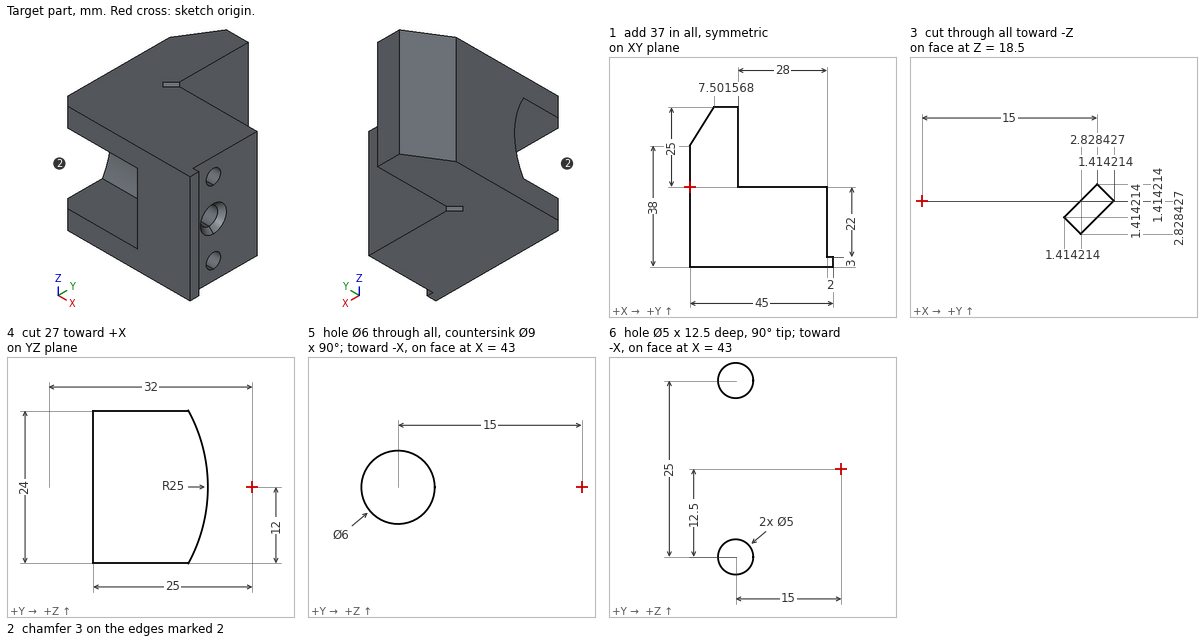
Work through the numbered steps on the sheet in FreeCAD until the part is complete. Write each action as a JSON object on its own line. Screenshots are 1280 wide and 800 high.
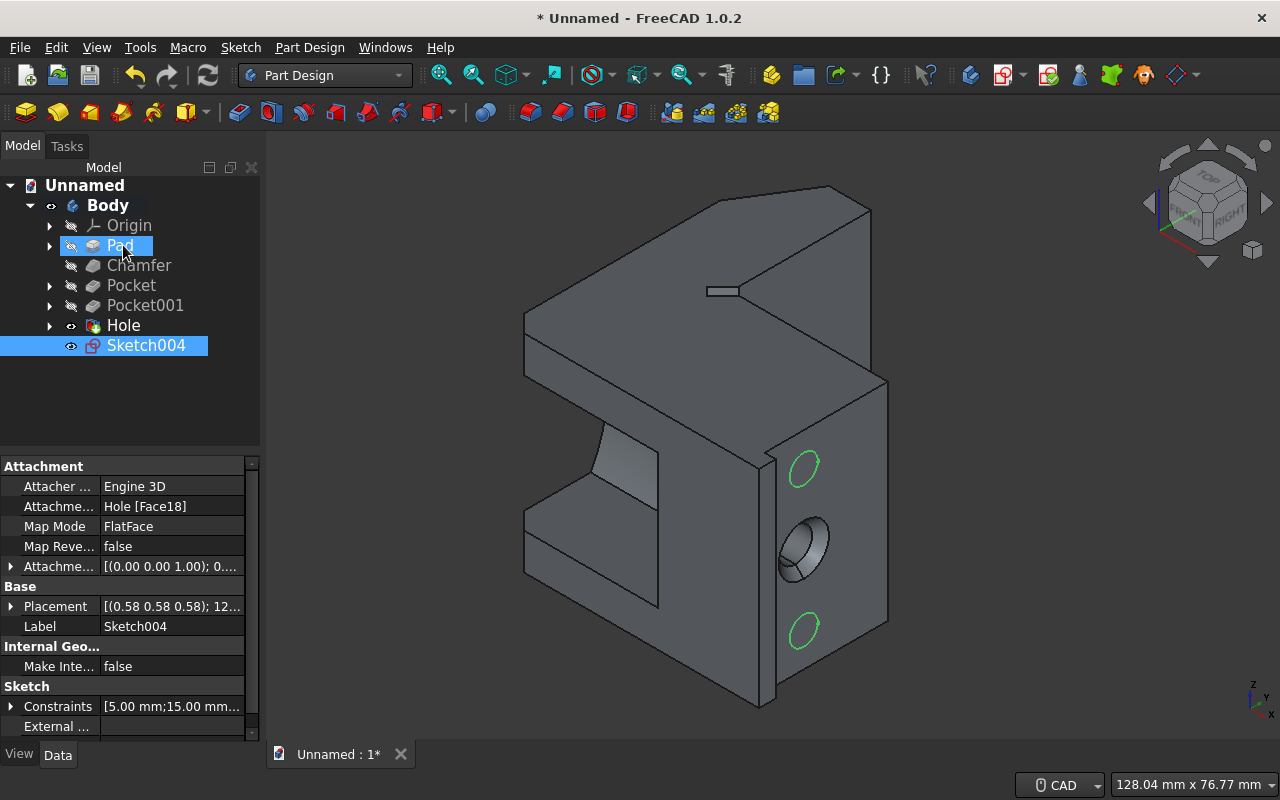
{"action": "left_click", "coordinate": [272, 112]}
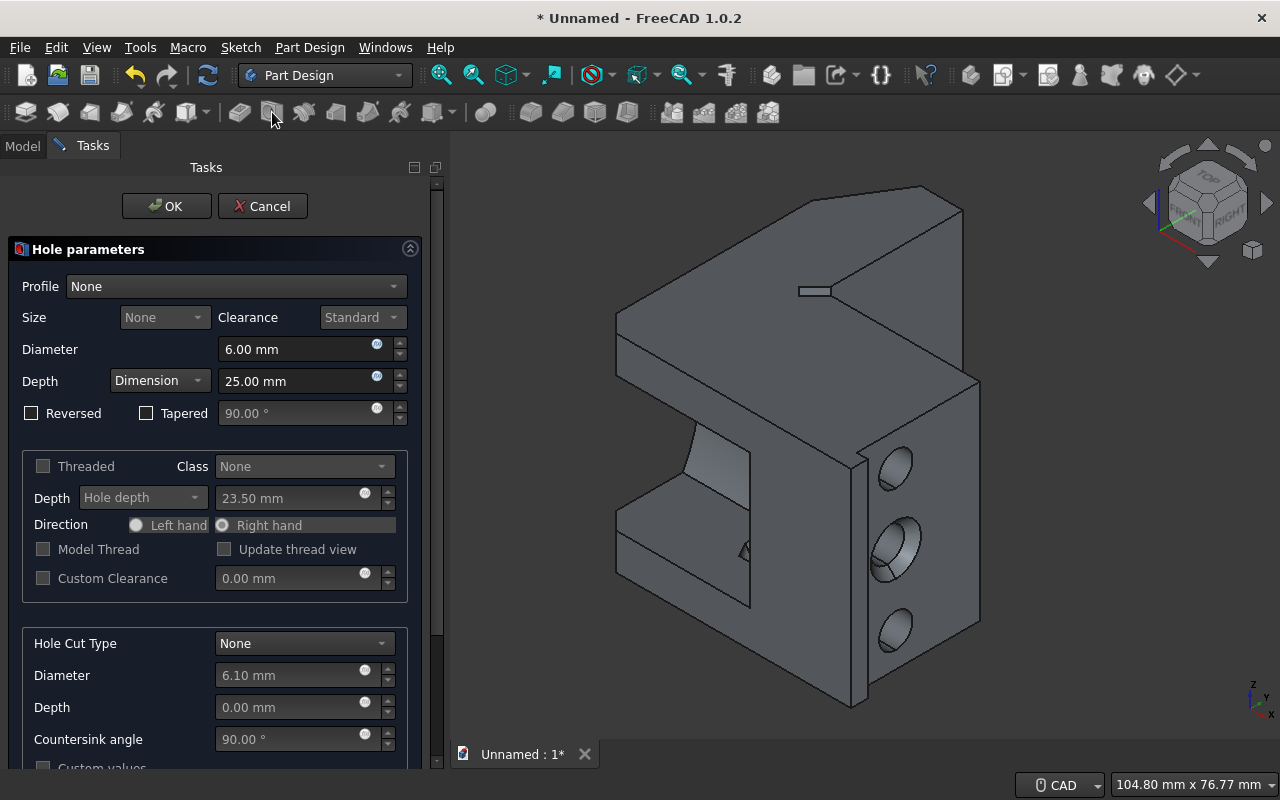
{"action": "triple_click", "coordinate": [305, 349]}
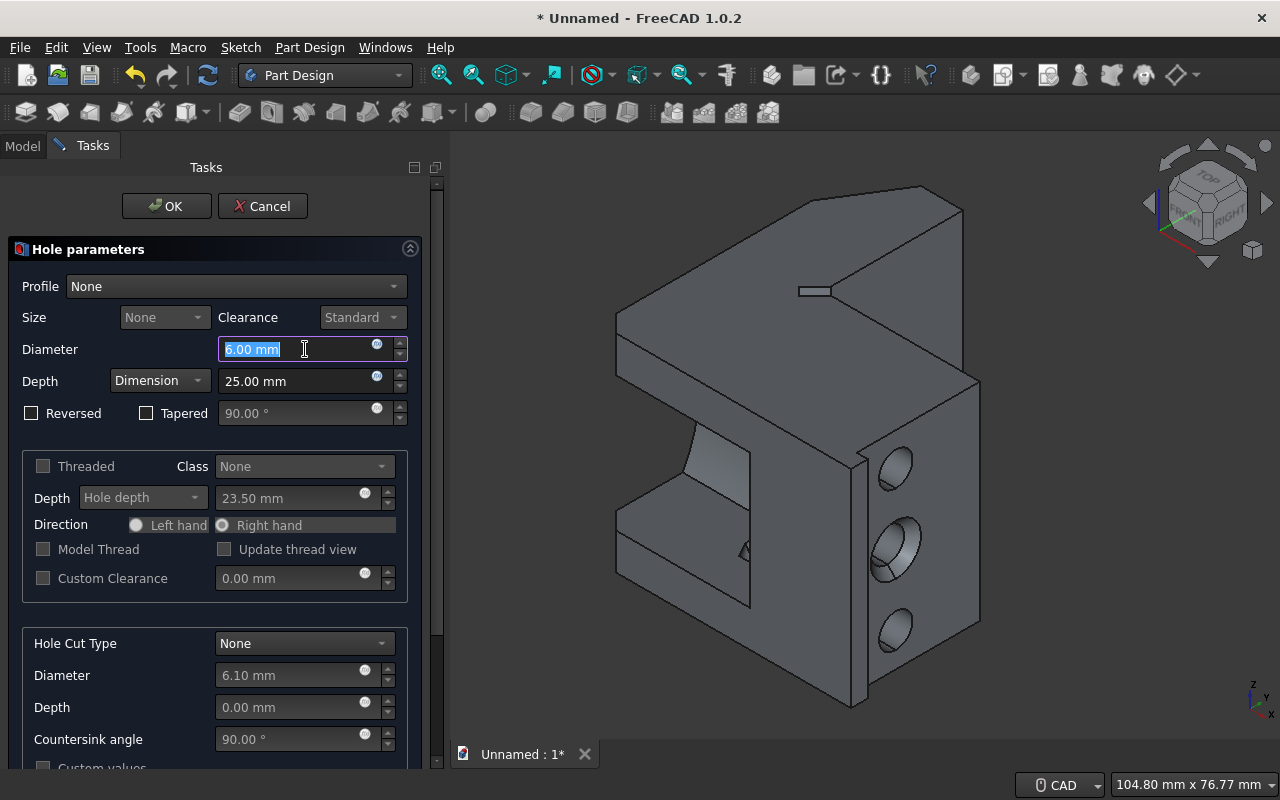
{"action": "type", "text": "5"}
{"action": "key", "text": "Tab"}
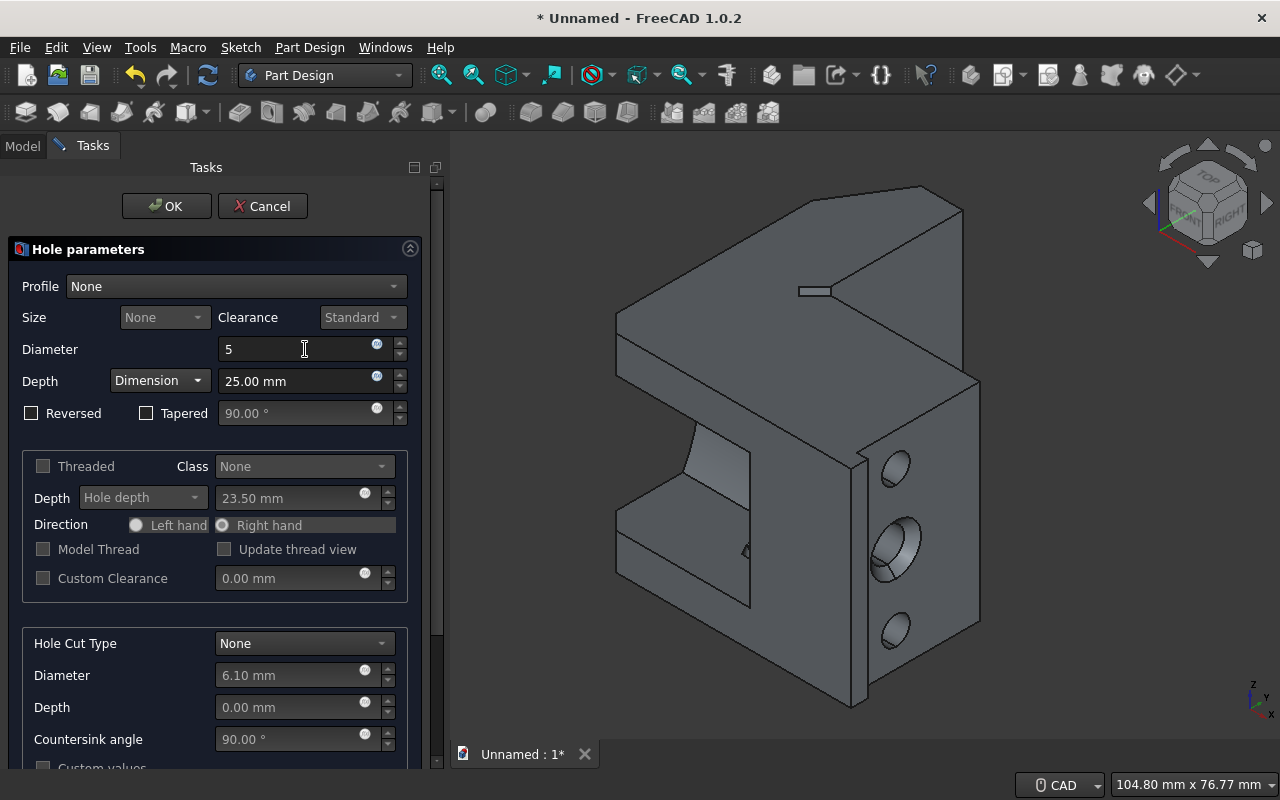
{"action": "triple_click", "coordinate": [305, 381]}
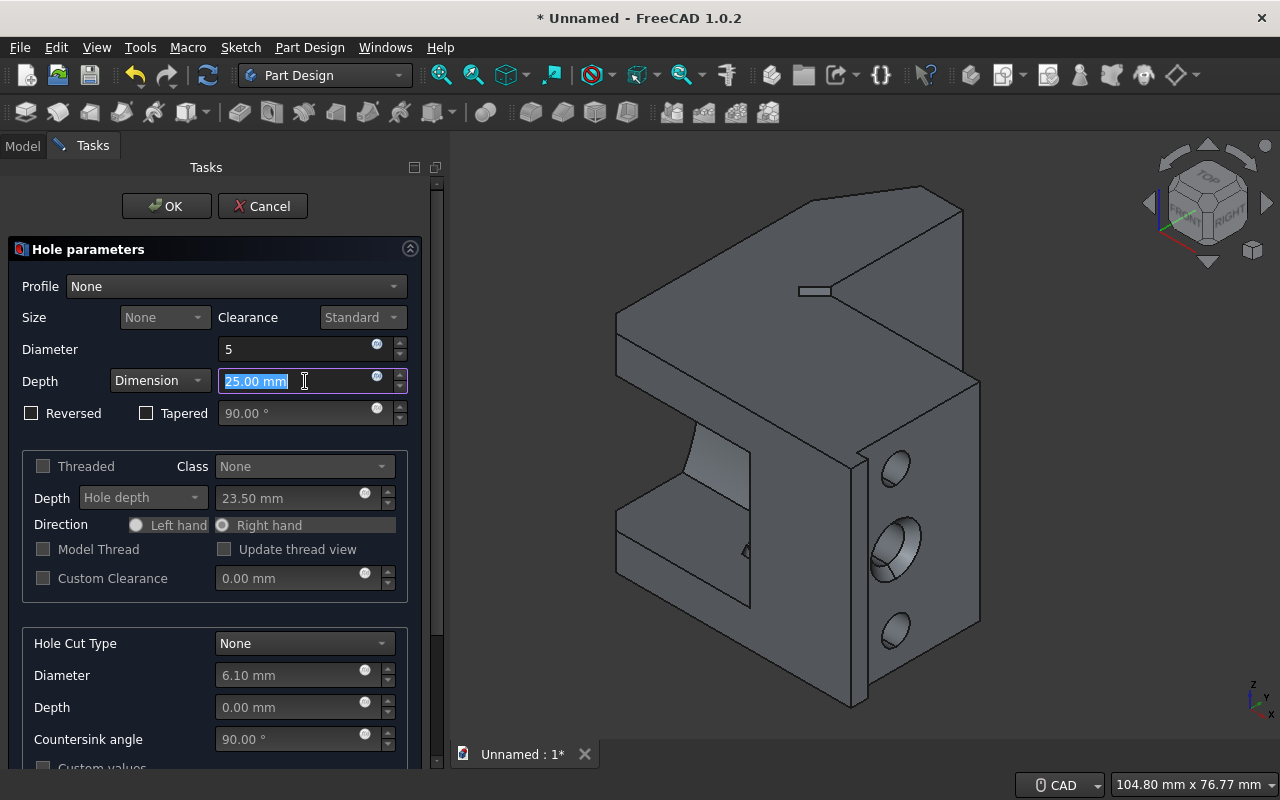
{"action": "type", "text": "12.5"}
{"action": "key", "text": "Tab"}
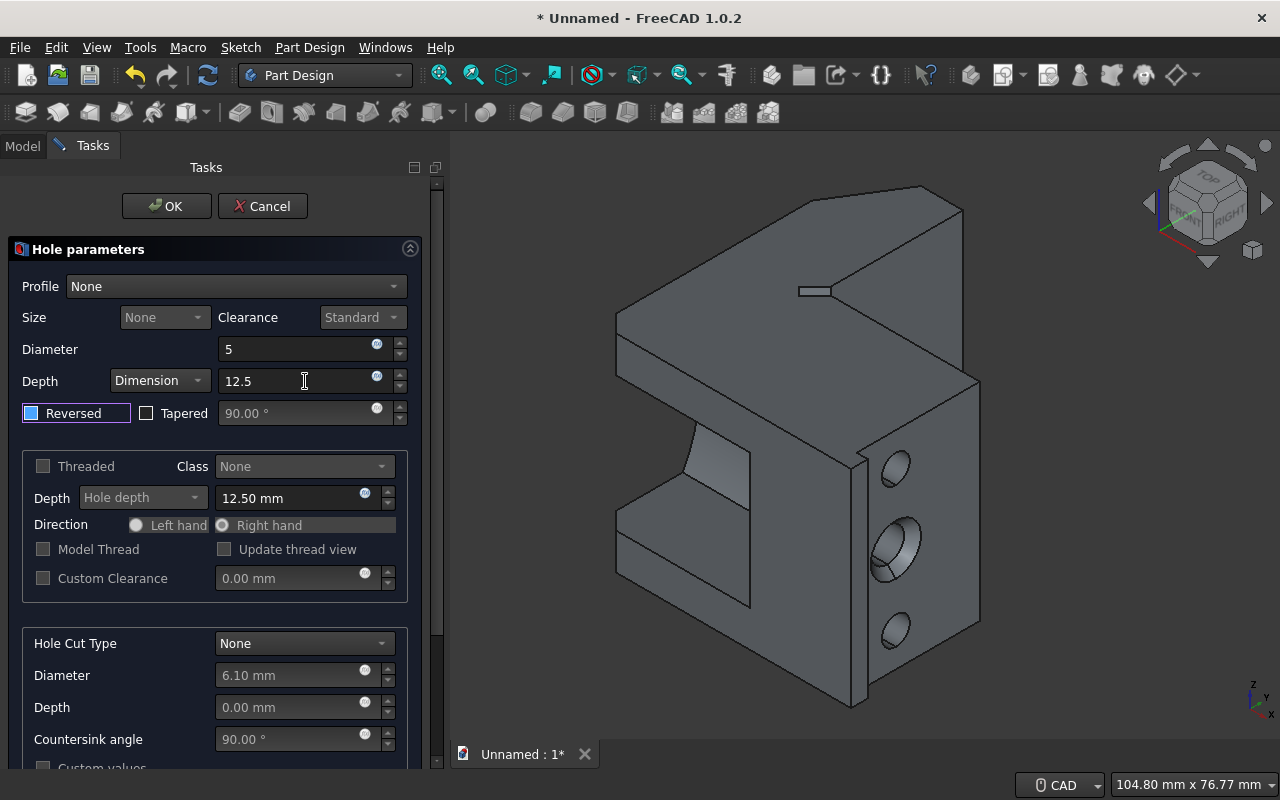
{"action": "scroll", "coordinate": [437, 472], "scroll_direction": "down", "scroll_amount": 3}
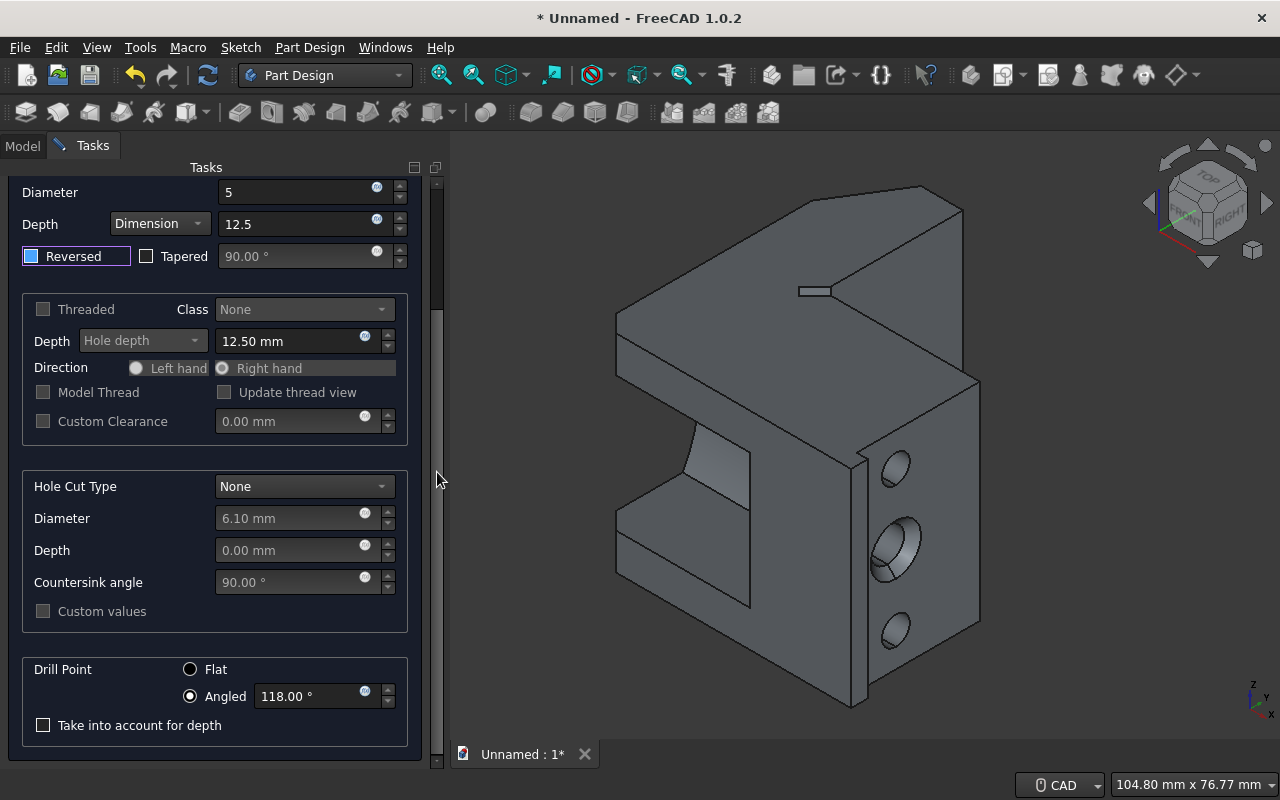
{"action": "triple_click", "coordinate": [317, 696]}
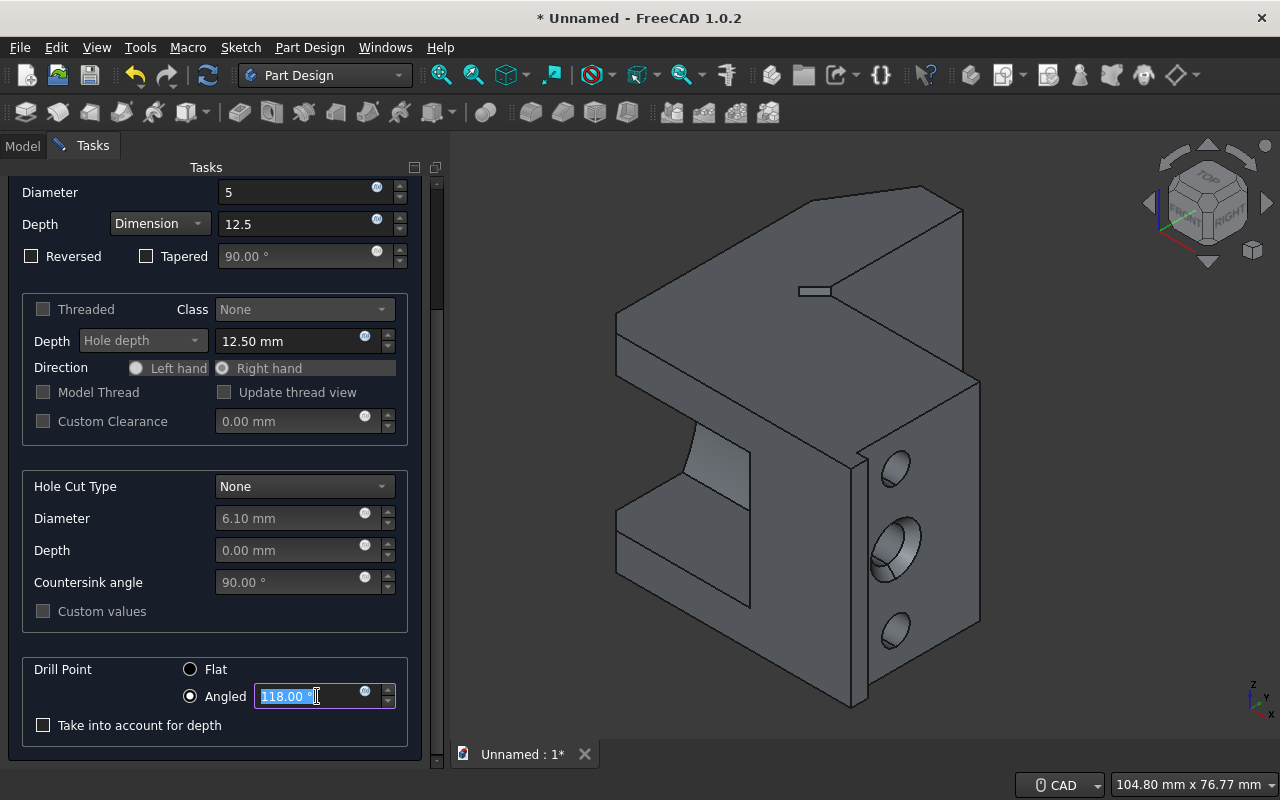
{"action": "type", "text": "90"}
{"action": "key", "text": "Tab"}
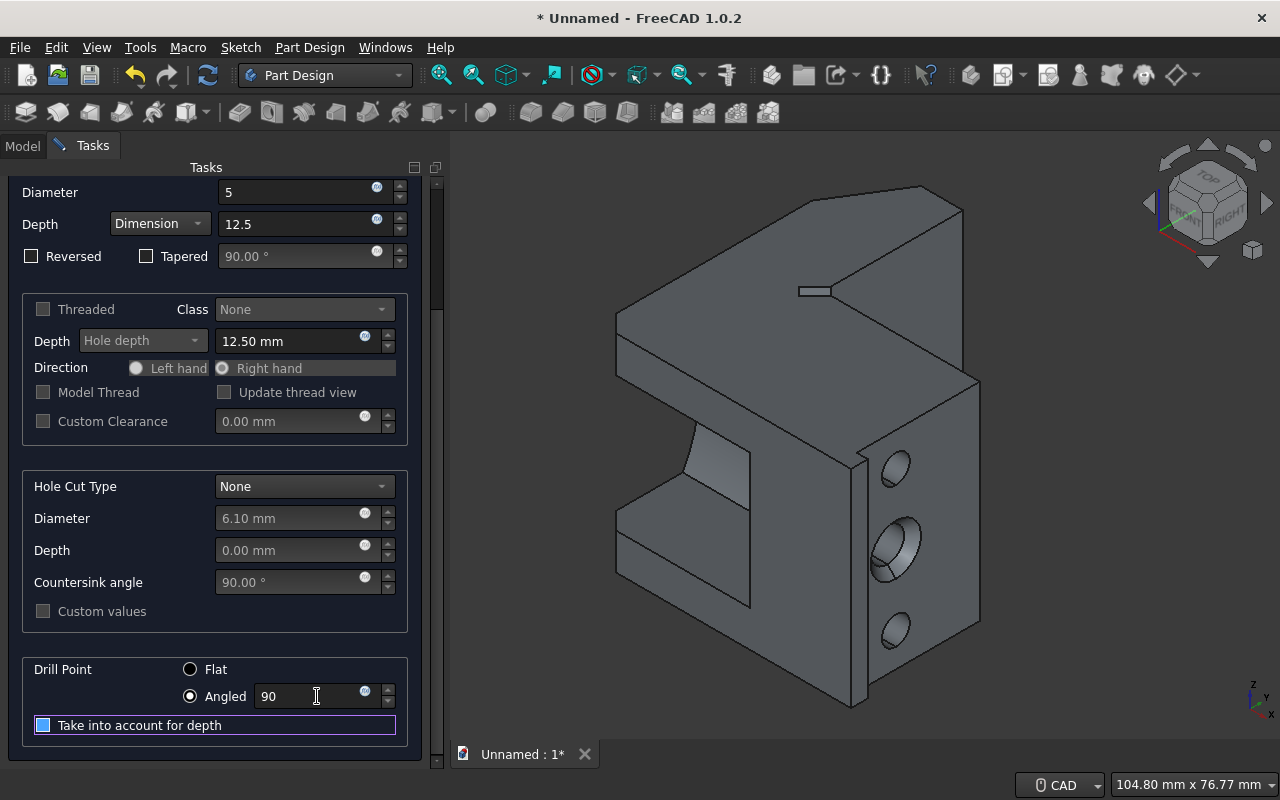
{"action": "scroll", "coordinate": [437, 472], "scroll_direction": "up", "scroll_amount": 4}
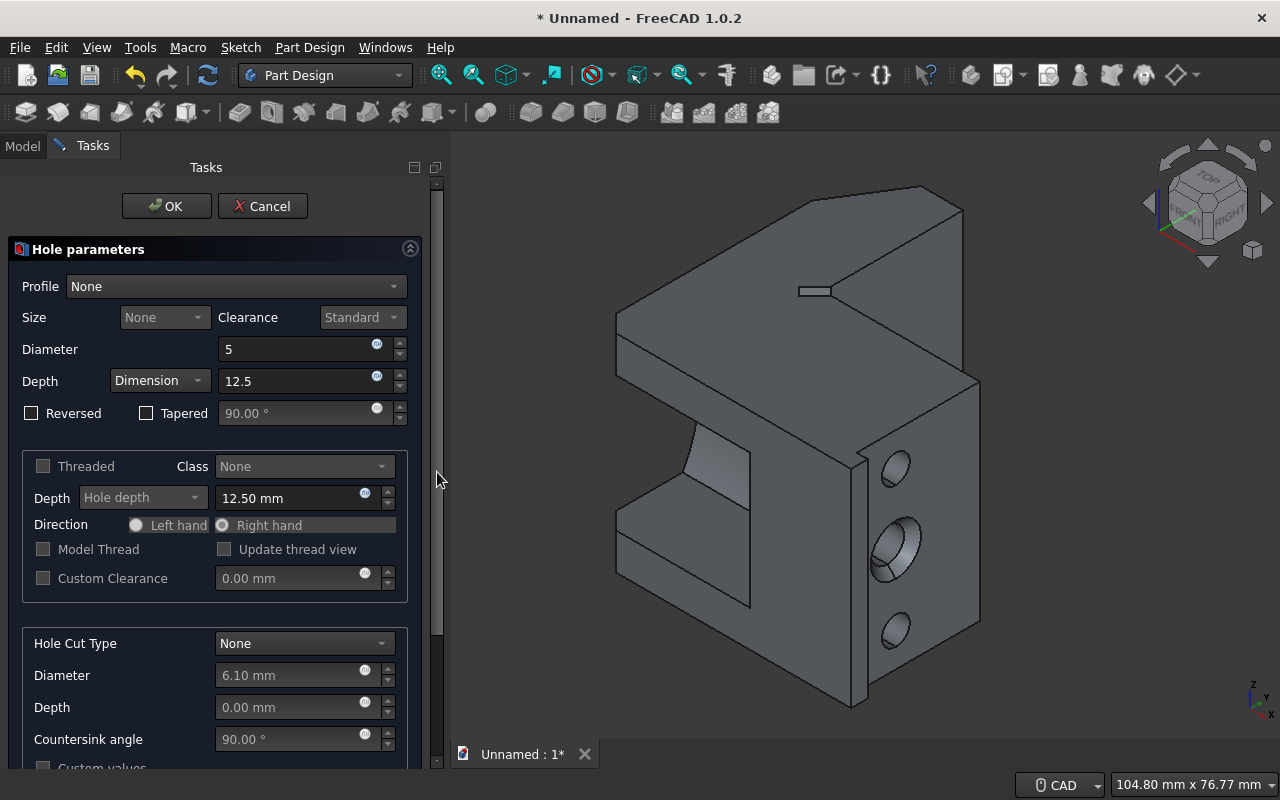
{"action": "left_click", "coordinate": [167, 206]}